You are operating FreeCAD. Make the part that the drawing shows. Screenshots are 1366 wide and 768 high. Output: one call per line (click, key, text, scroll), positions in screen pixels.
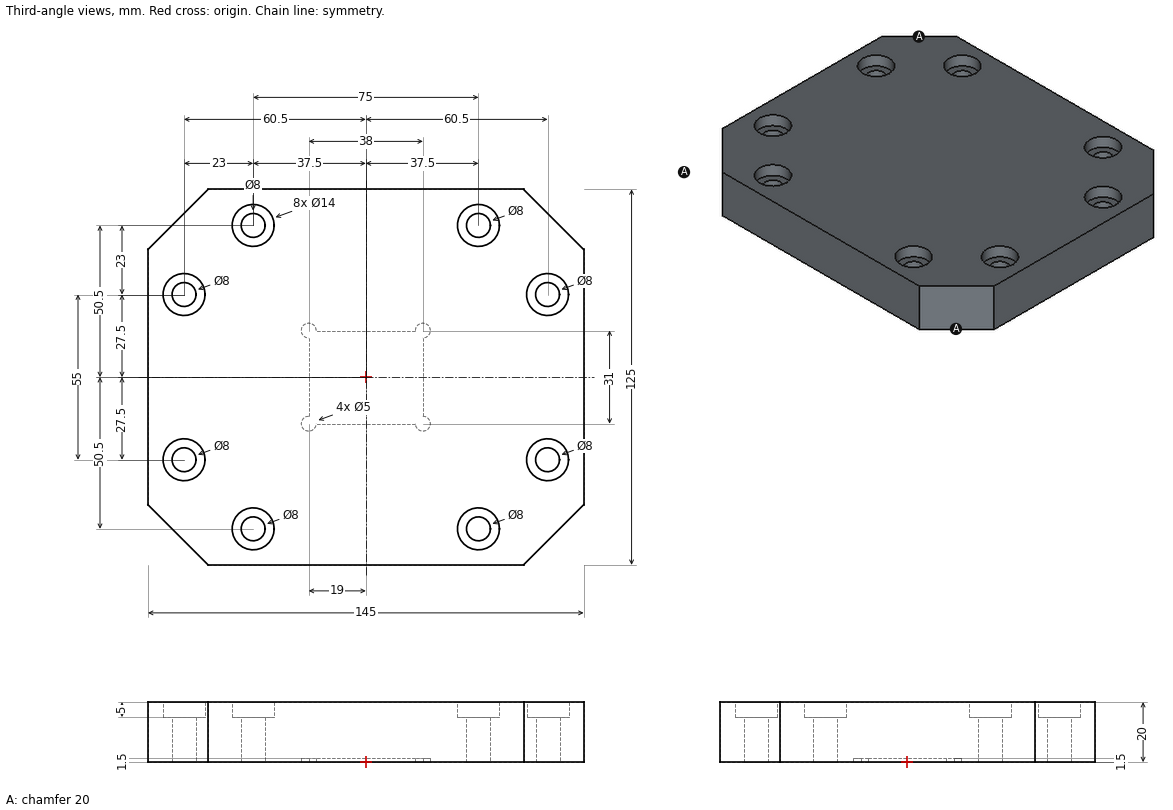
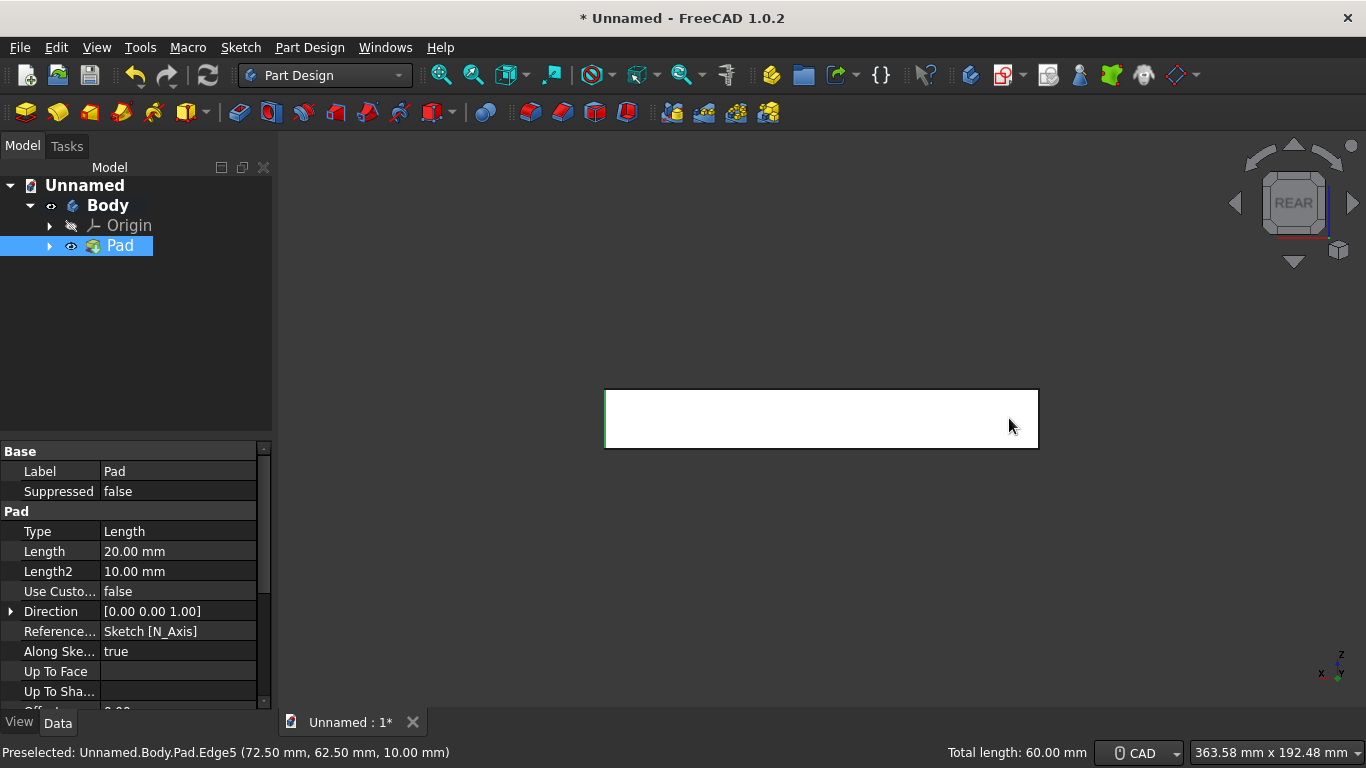
click(442, 76)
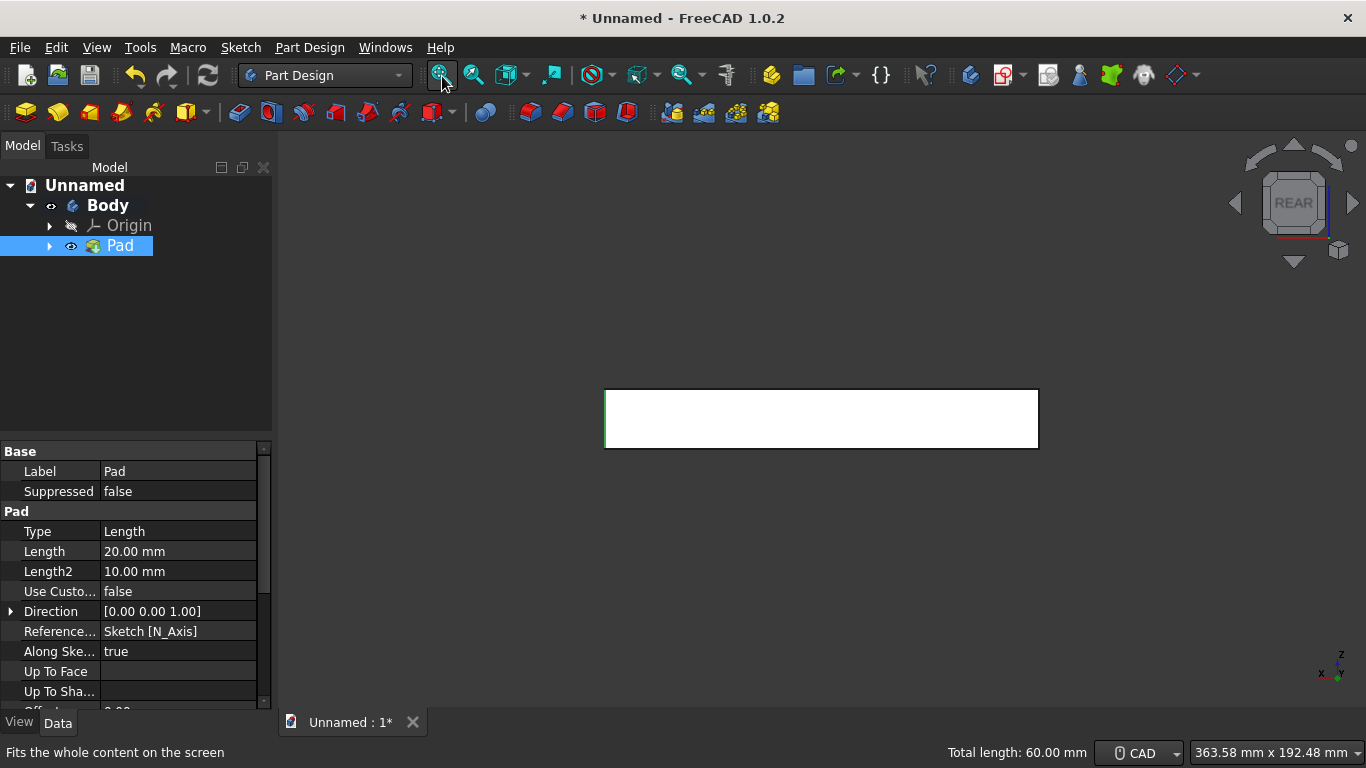
click(1039, 418, ctrl)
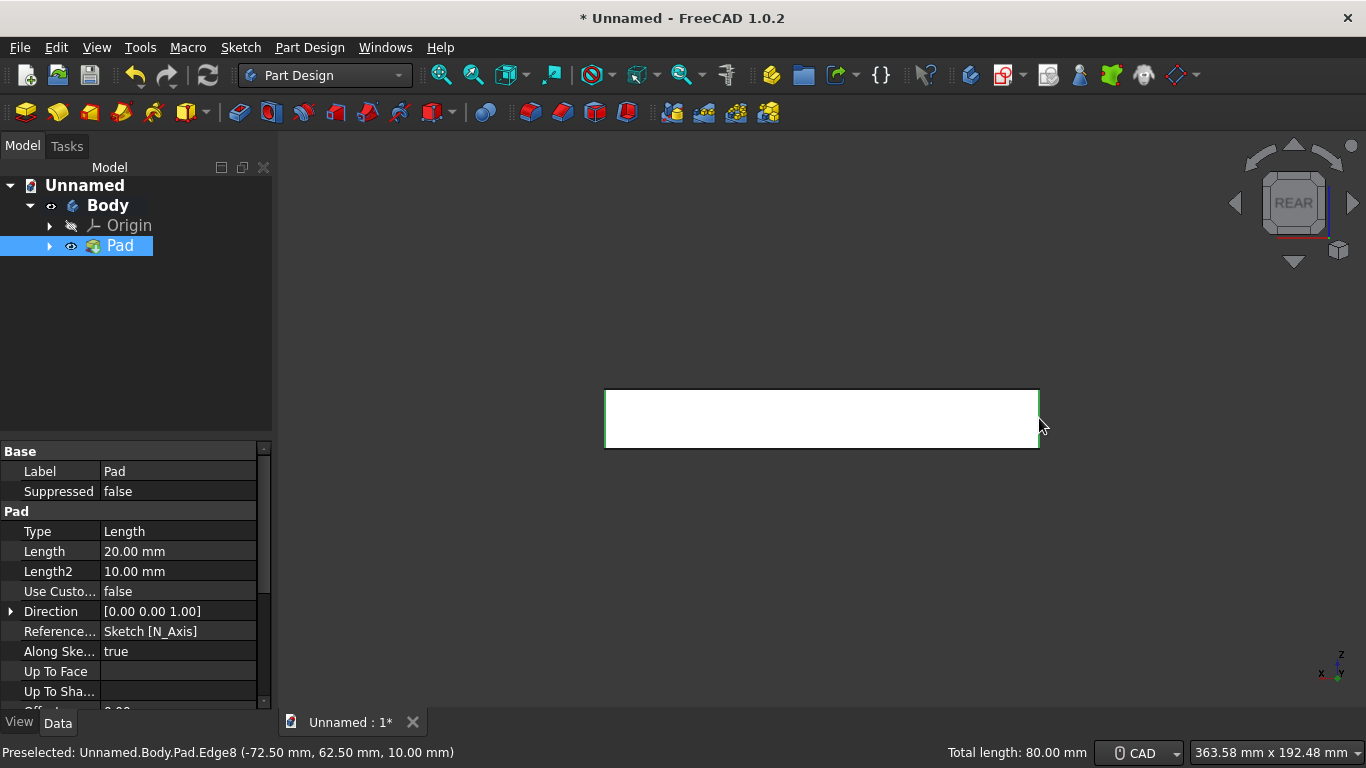
click(564, 112)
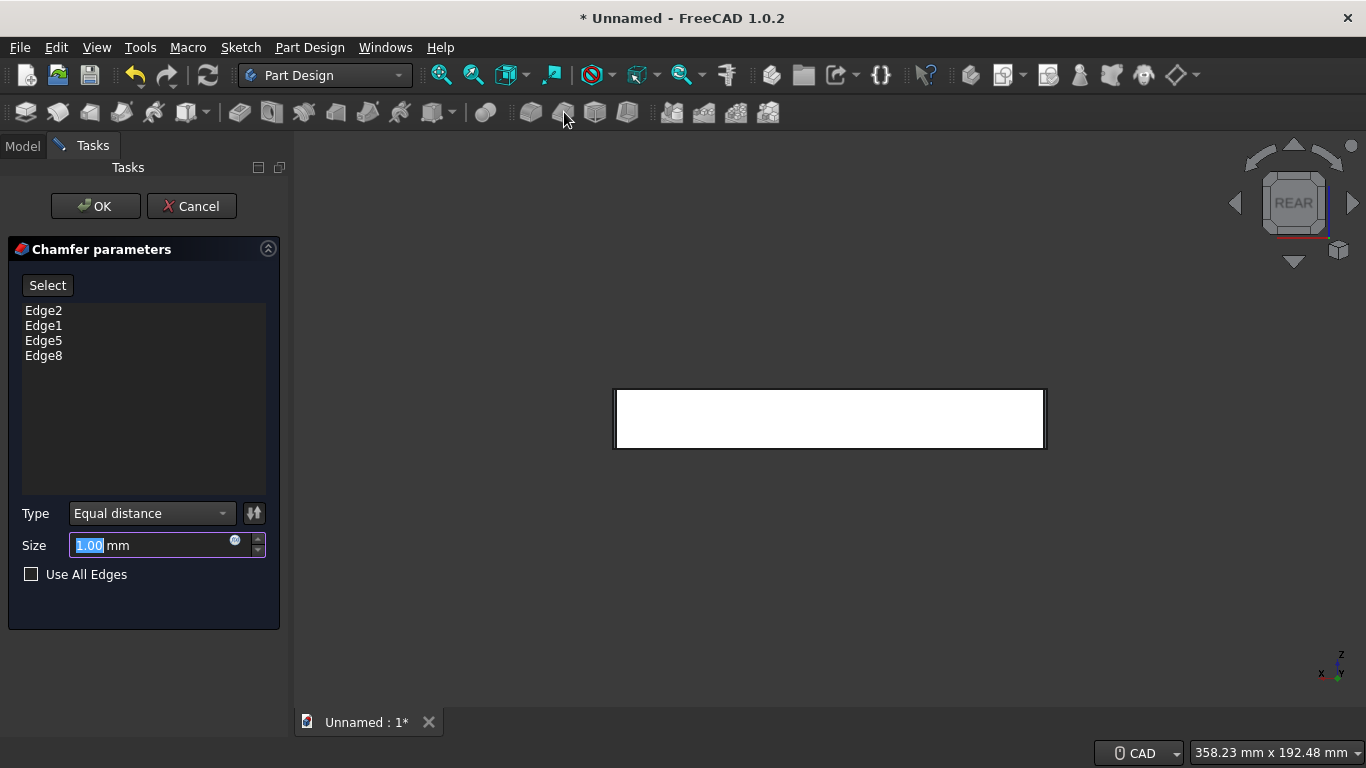
text(20)
key(Tab)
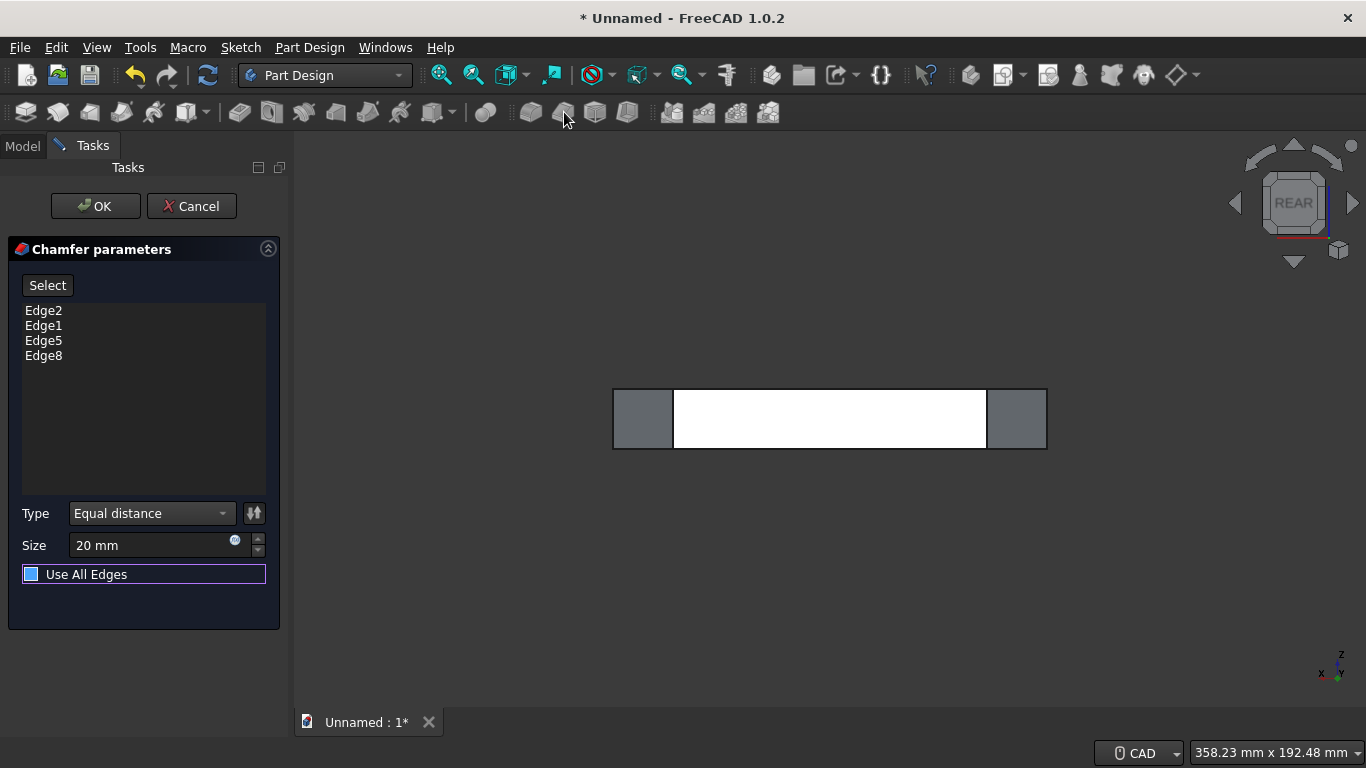
click(96, 206)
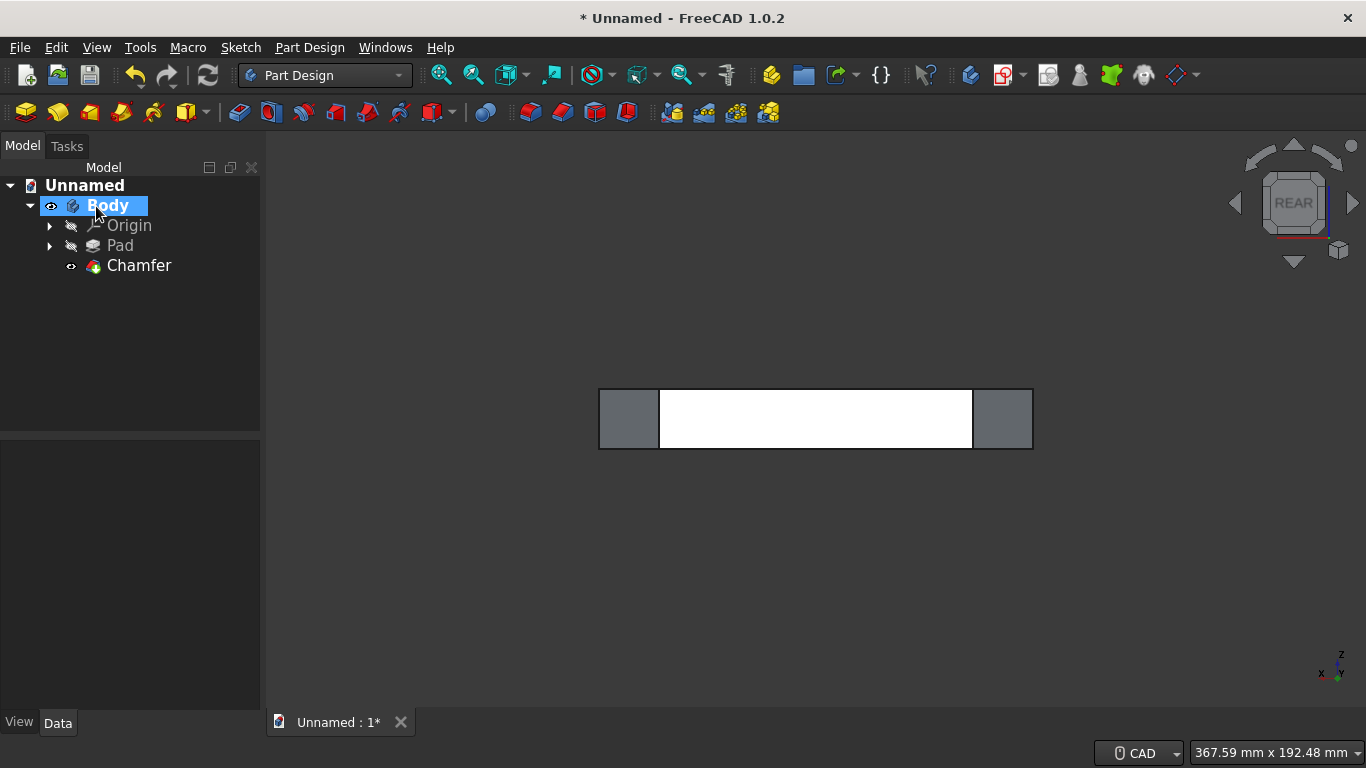
click(442, 76)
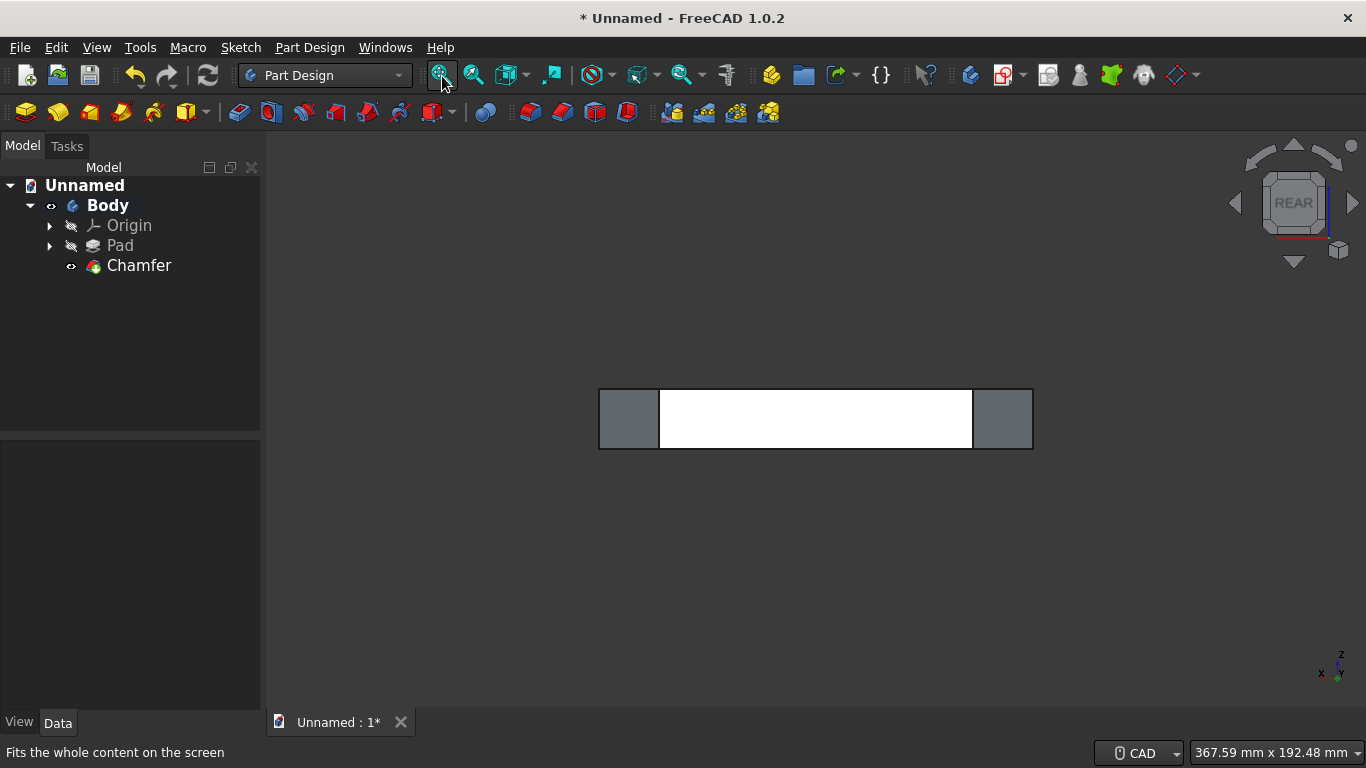
key(0)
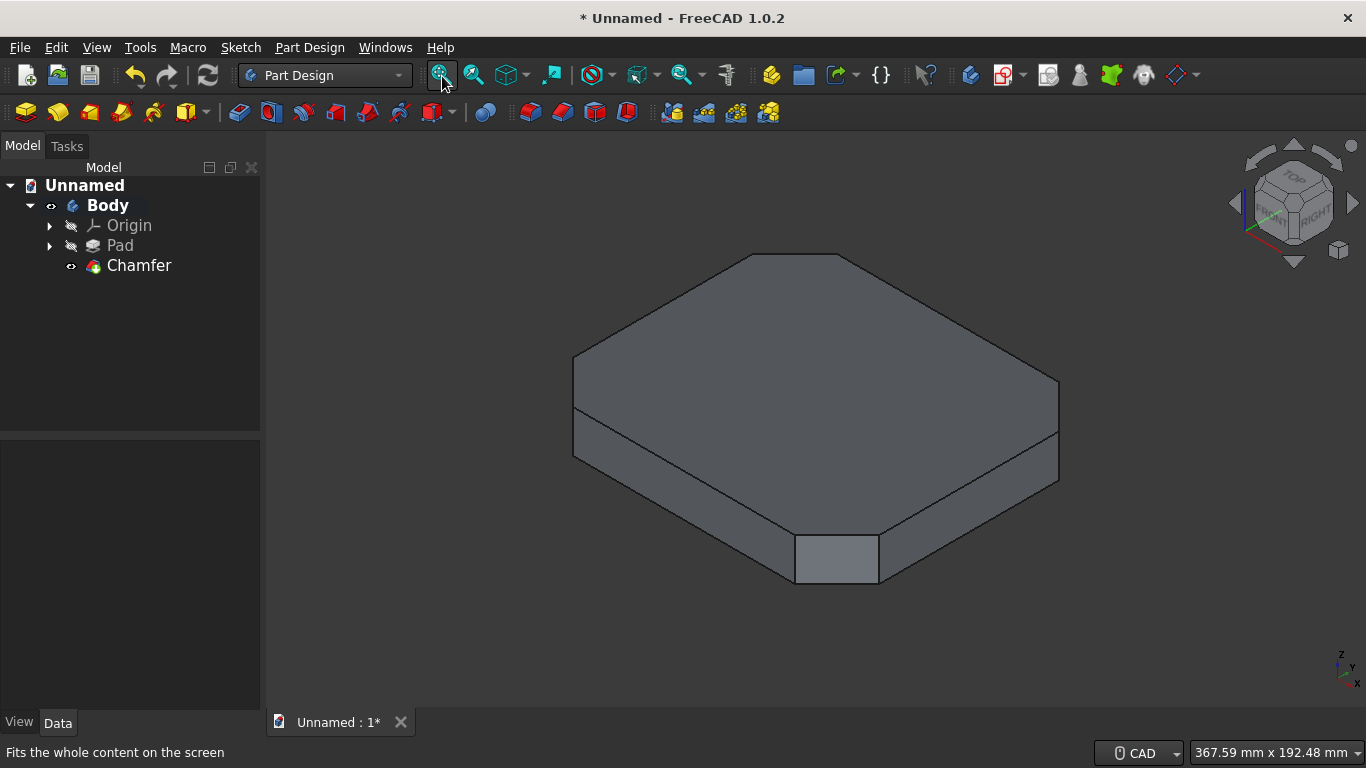
click(816, 394)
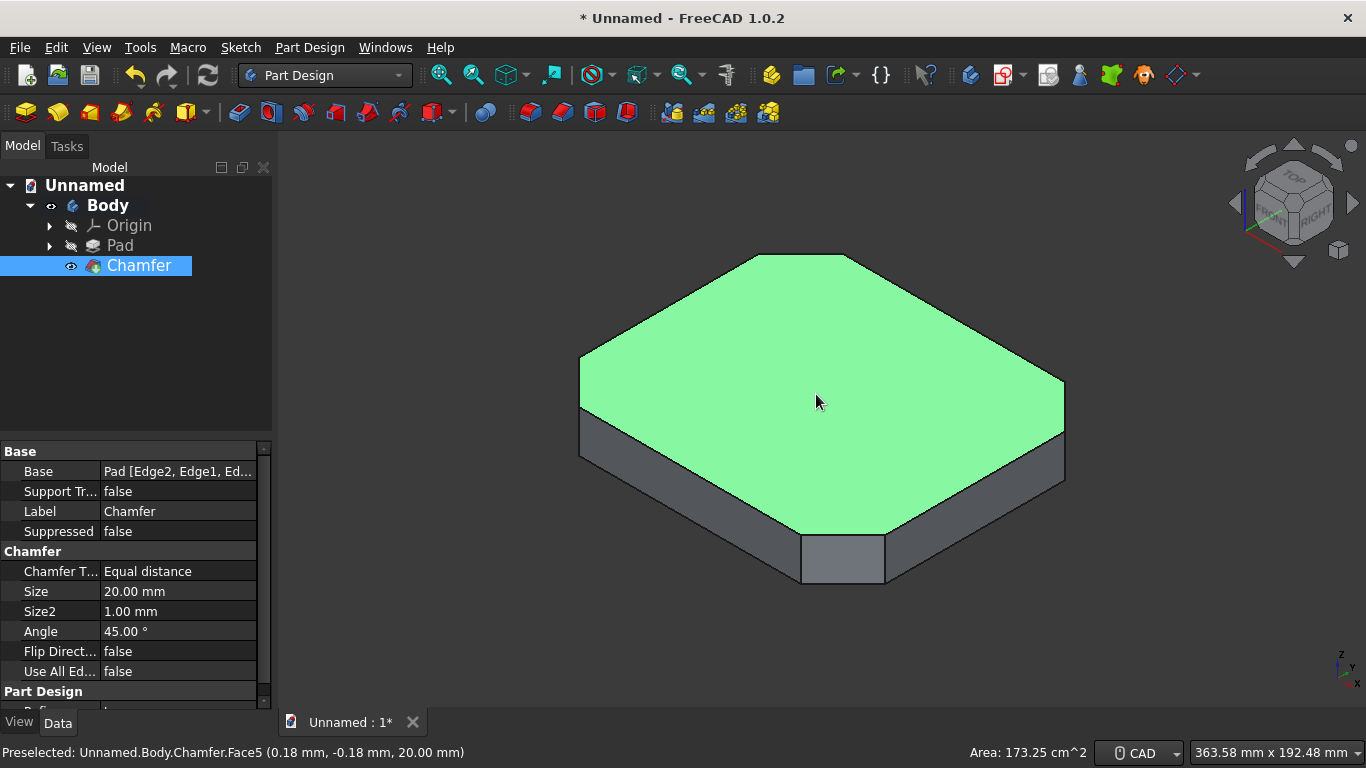
click(1004, 76)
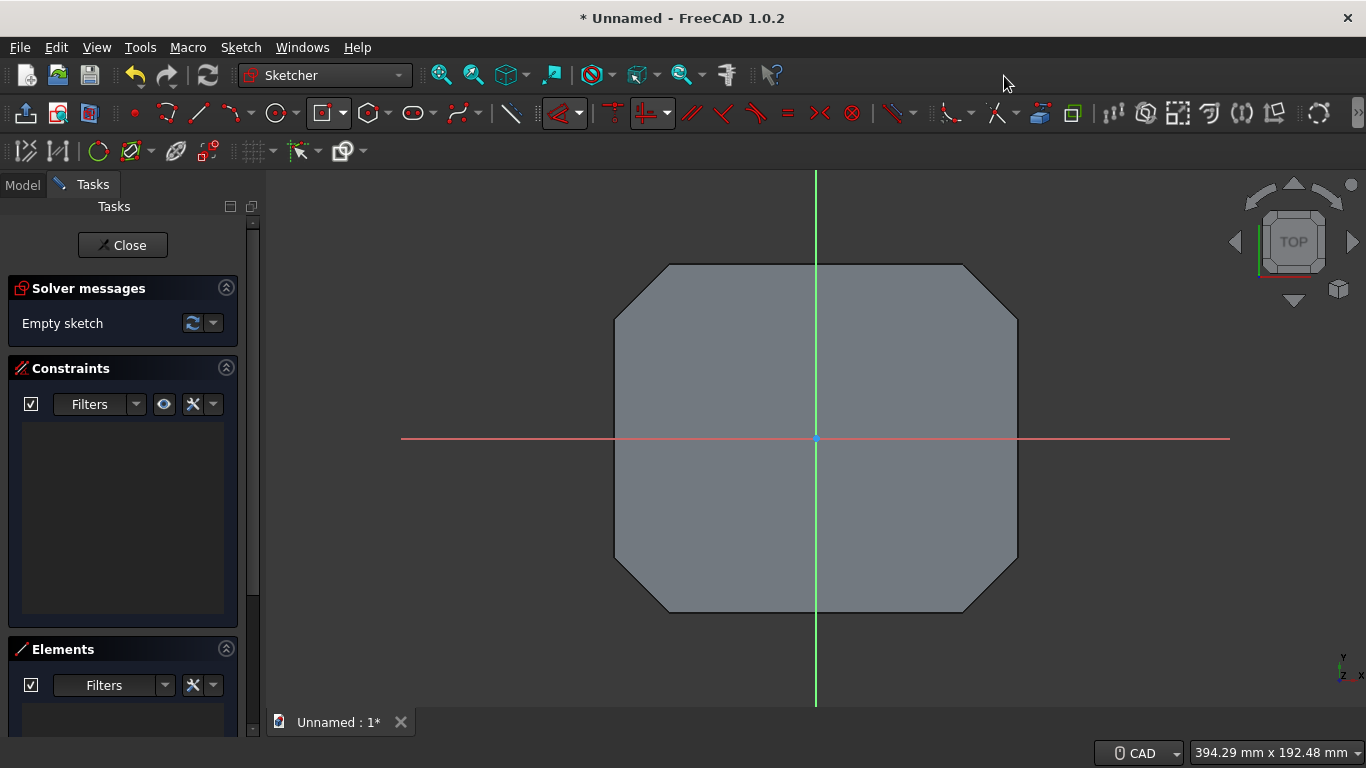
key(g)
key(c)